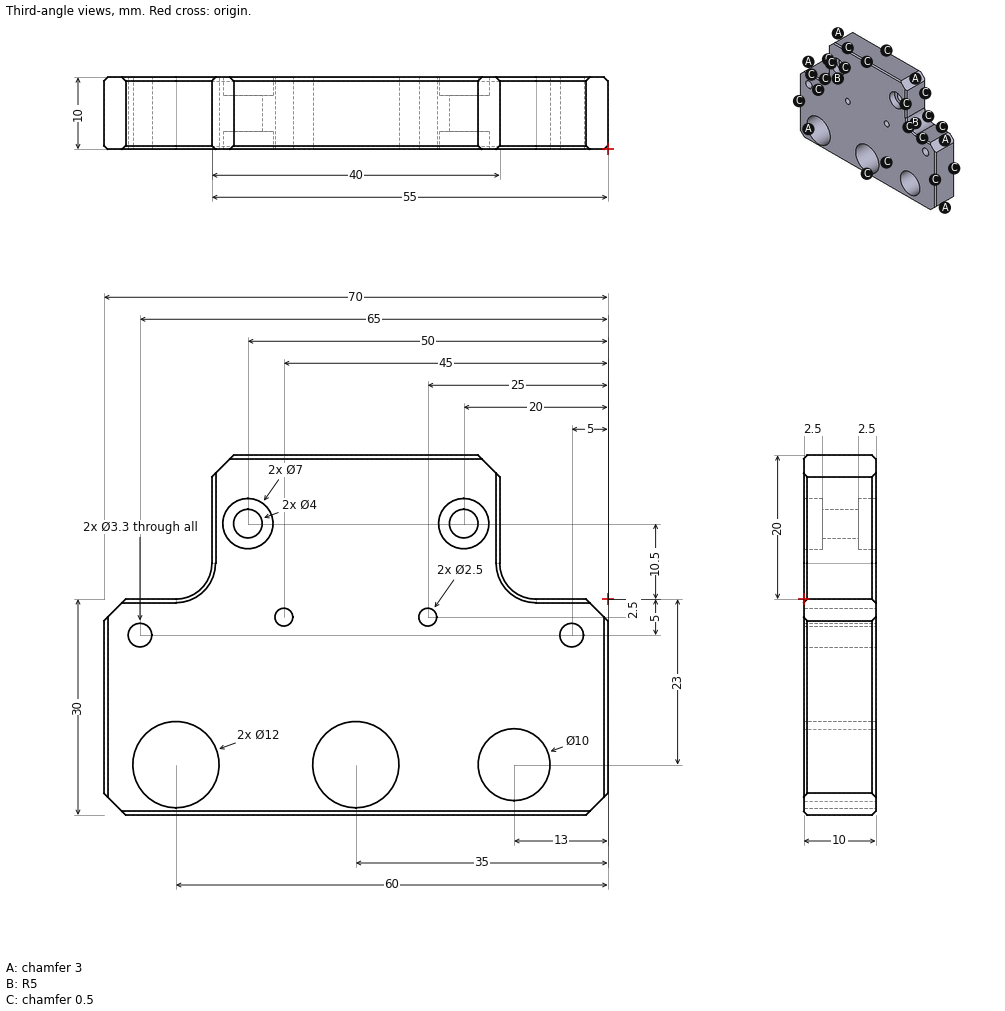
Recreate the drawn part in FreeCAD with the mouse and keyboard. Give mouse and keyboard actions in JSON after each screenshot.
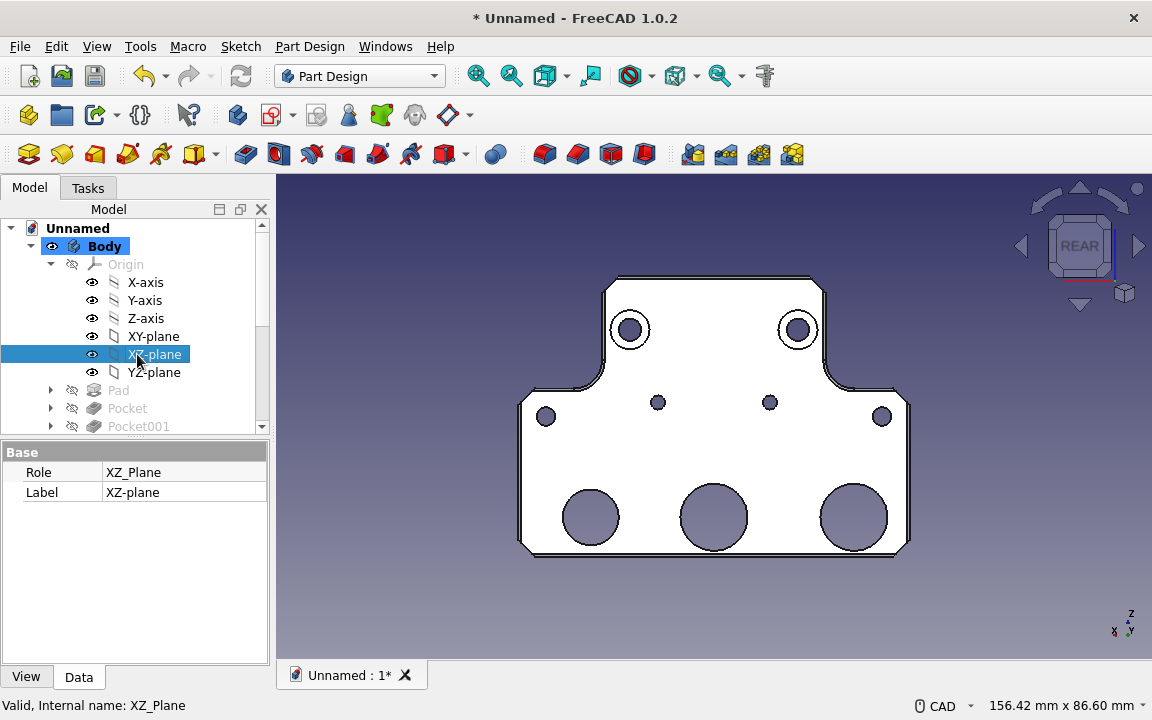
{"action": "left_click", "coordinate": [448, 116]}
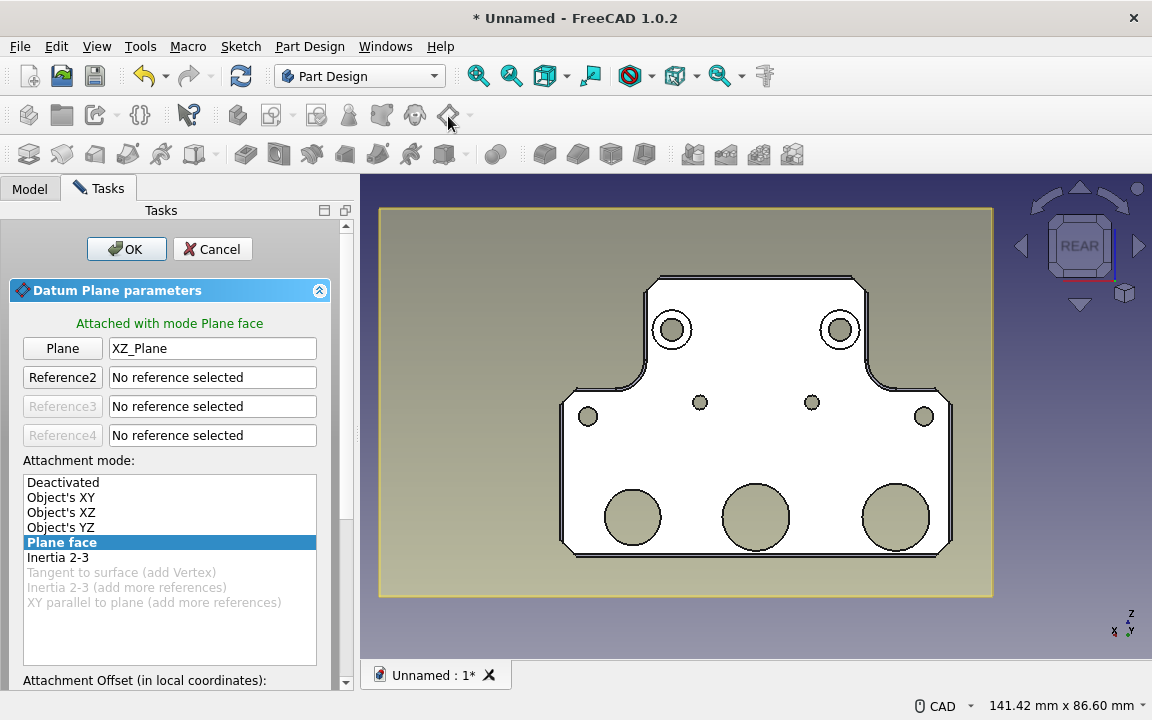
{"action": "scroll", "coordinate": [346, 455], "scroll_direction": "down", "scroll_amount": 3}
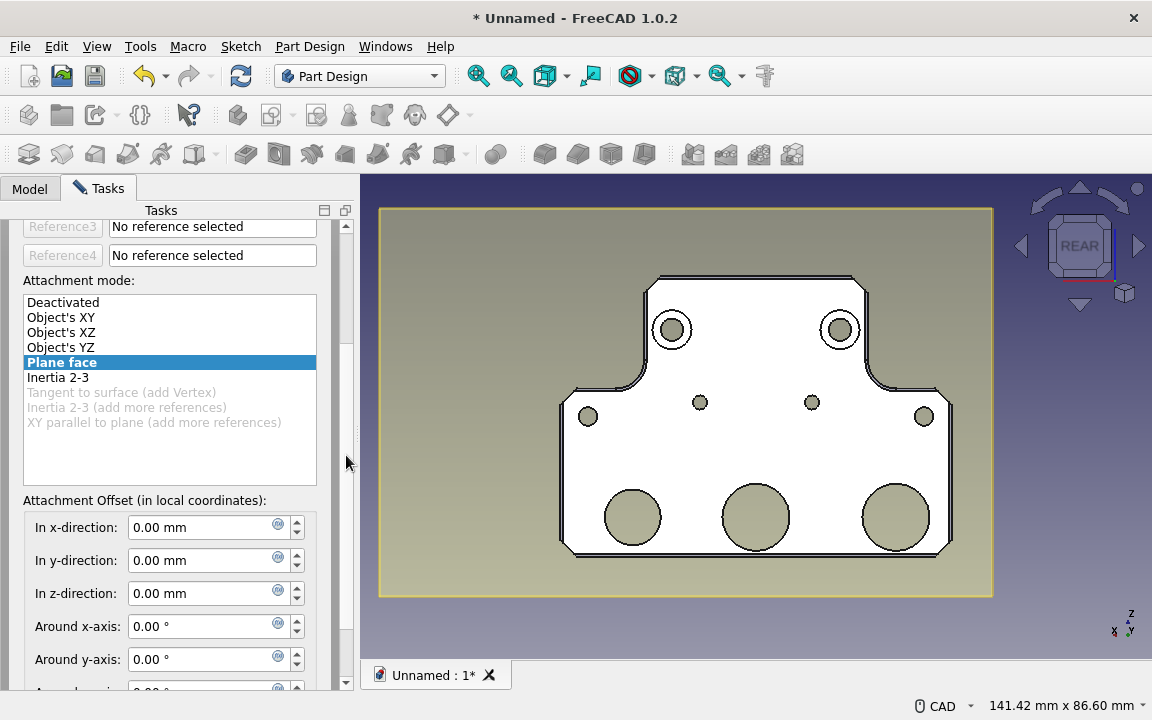
{"action": "triple_click", "coordinate": [210, 594]}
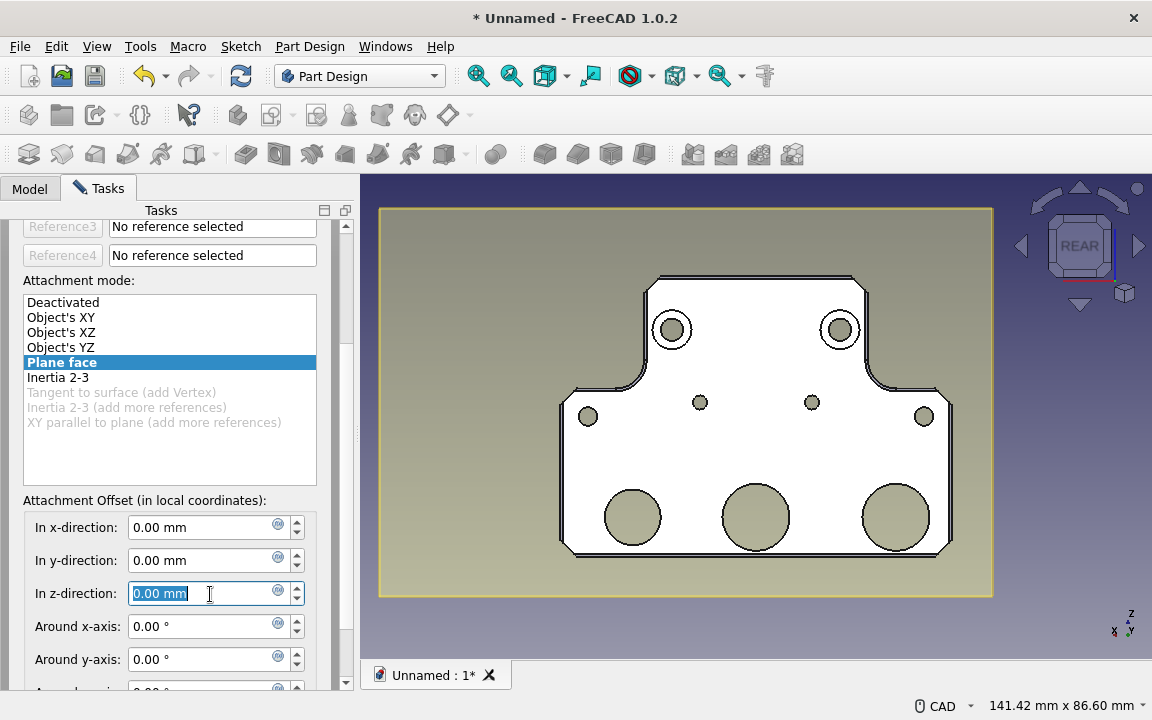
{"action": "type", "text": "-2.5"}
{"action": "key", "text": "Tab"}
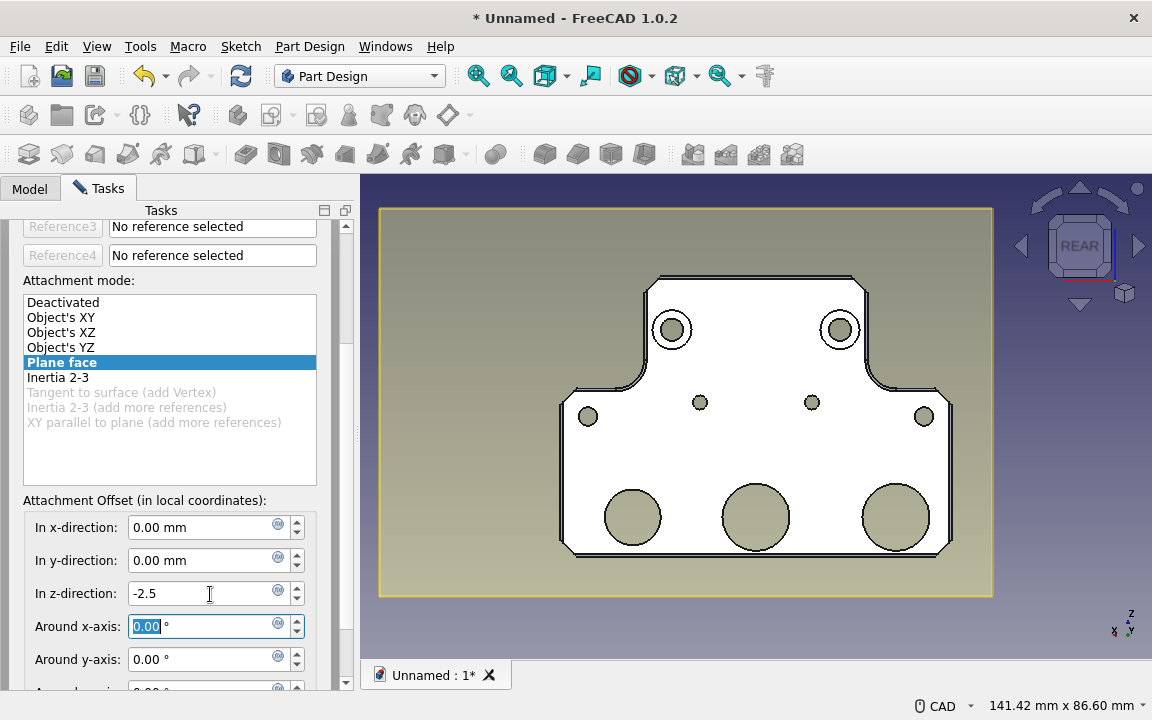
{"action": "scroll", "coordinate": [346, 455], "scroll_direction": "up", "scroll_amount": 4}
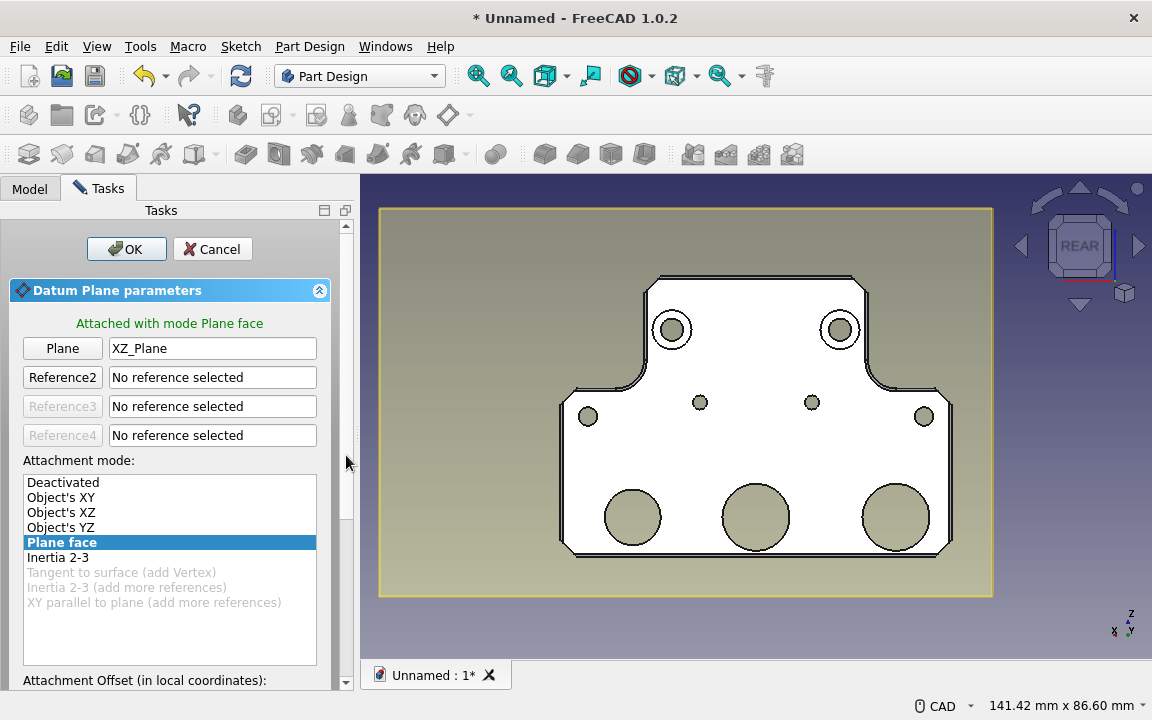
{"action": "left_click", "coordinate": [127, 249]}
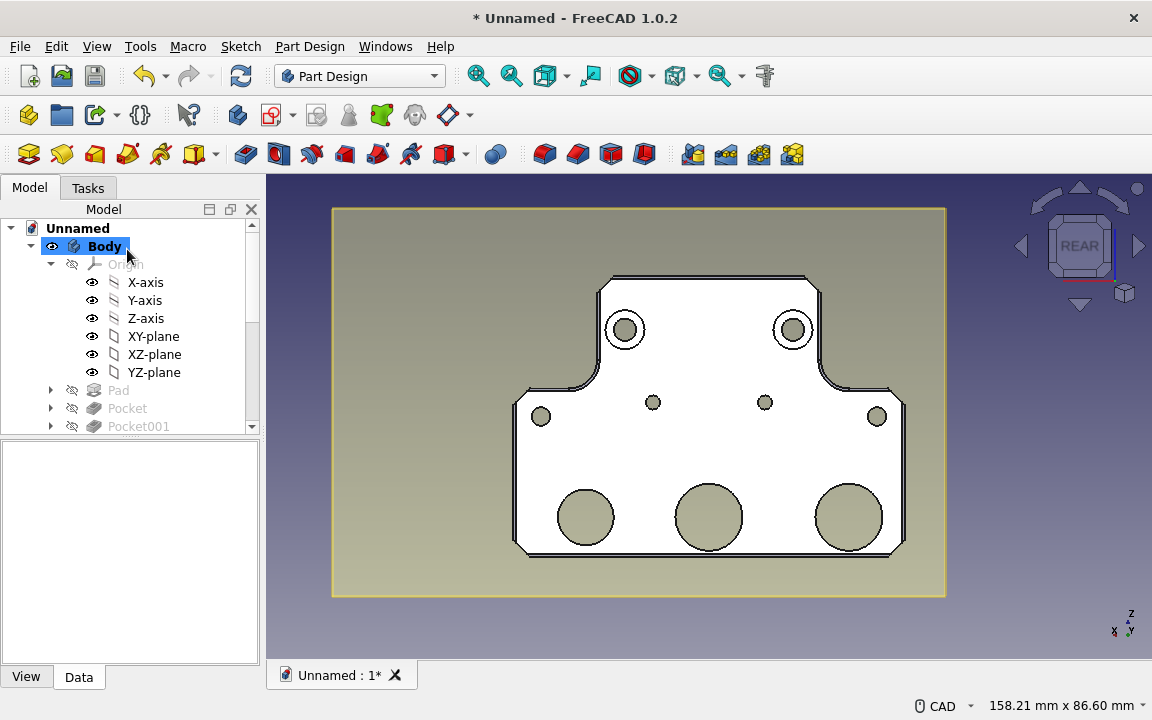
{"action": "scroll", "coordinate": [101, 332], "scroll_direction": "down", "scroll_amount": 3}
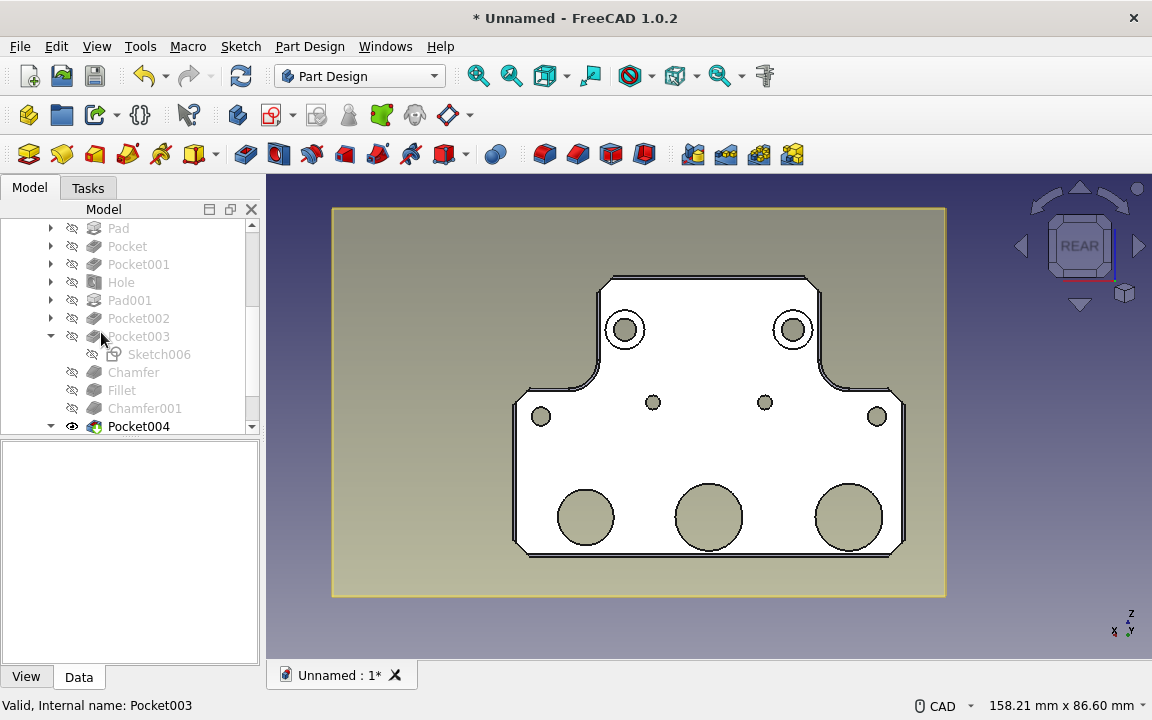
{"action": "scroll", "coordinate": [141, 332], "scroll_direction": "up", "scroll_amount": 15}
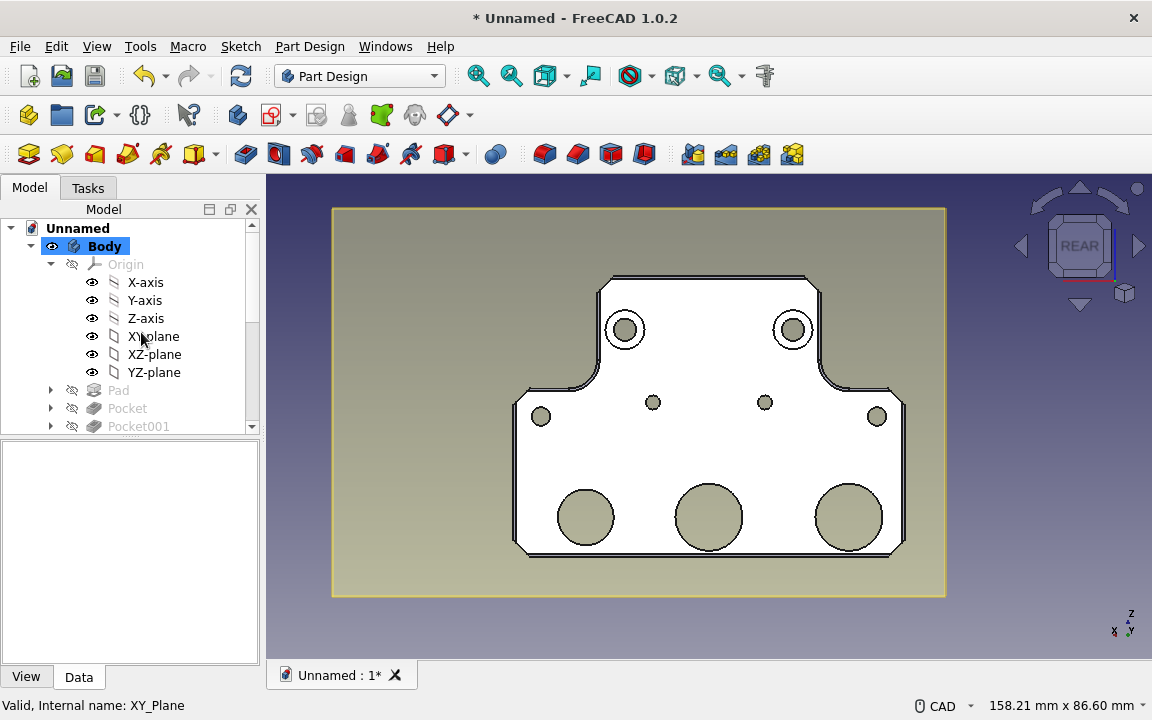
{"action": "scroll", "coordinate": [101, 332], "scroll_direction": "down", "scroll_amount": 6}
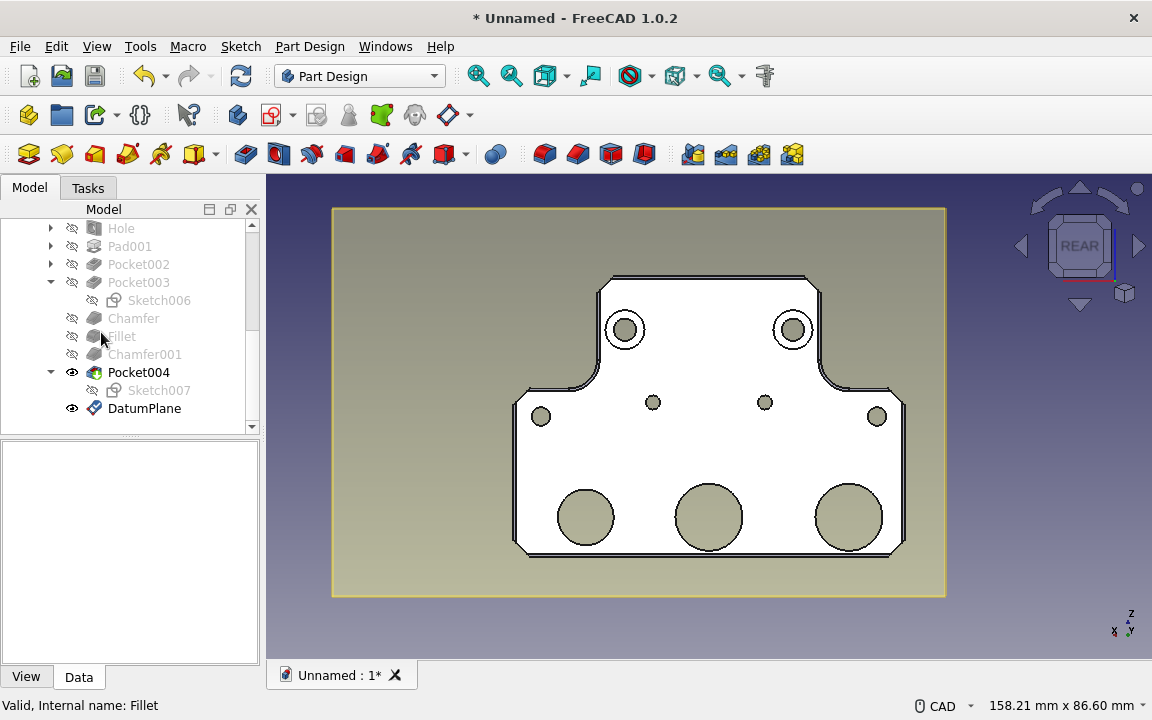
{"action": "left_click", "coordinate": [117, 408]}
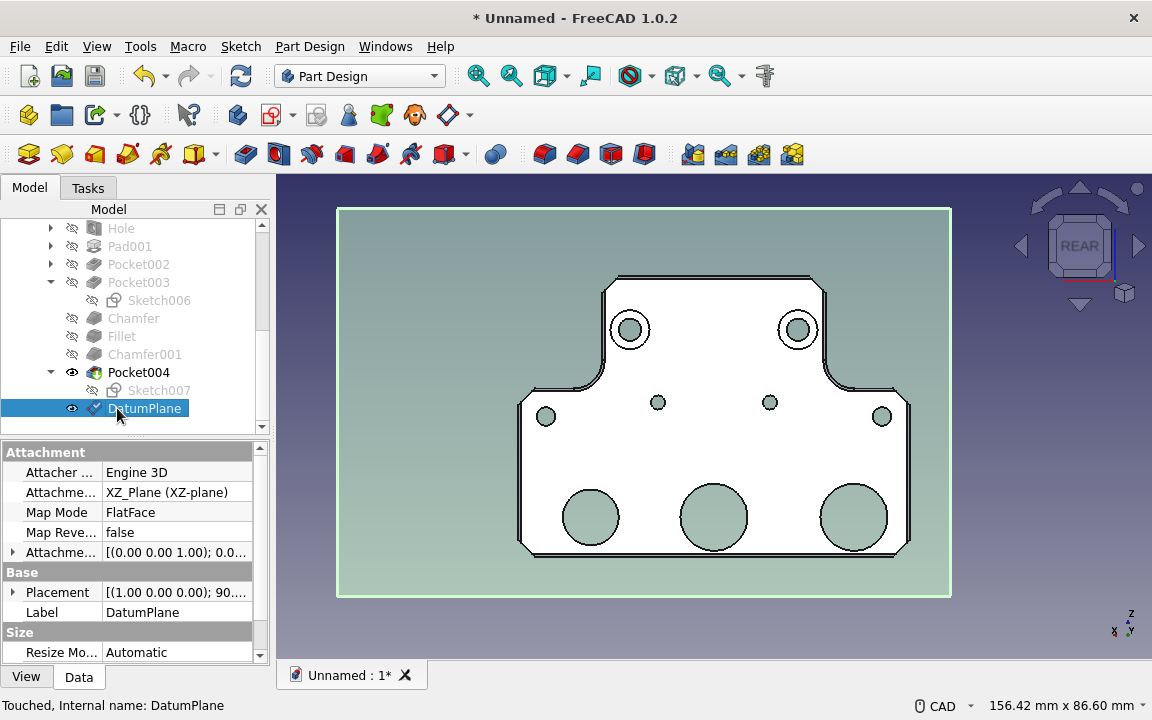
{"action": "left_click", "coordinate": [270, 116]}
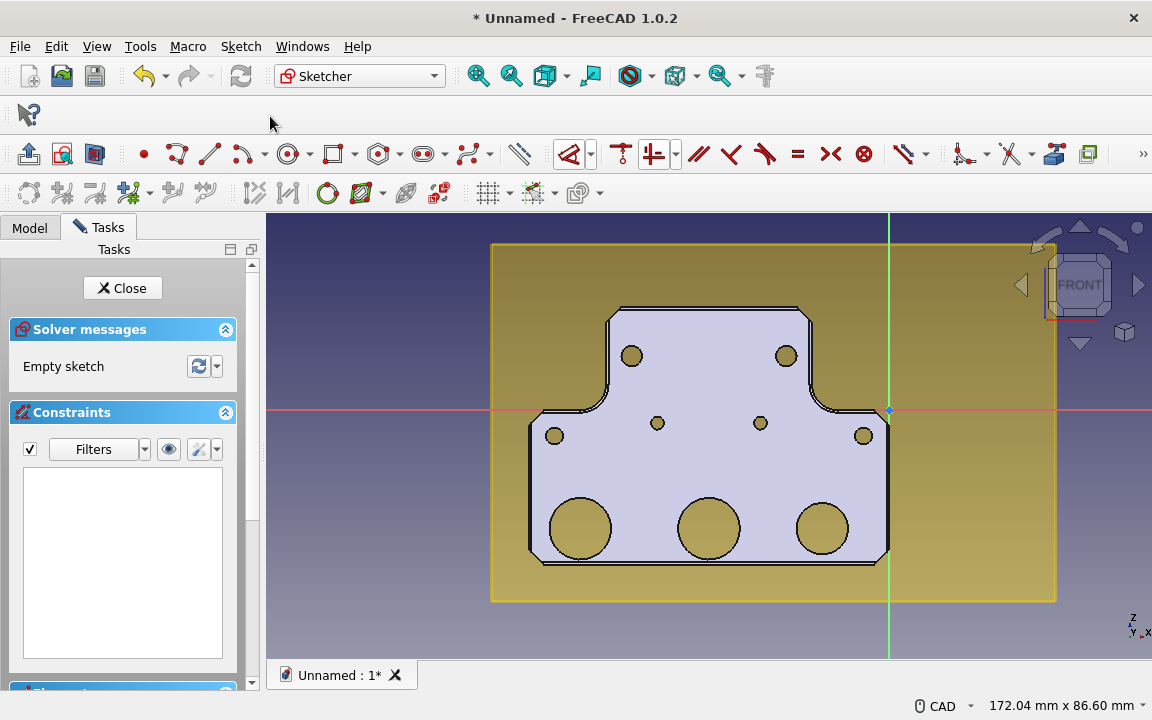
{"action": "left_click", "coordinate": [95, 154]}